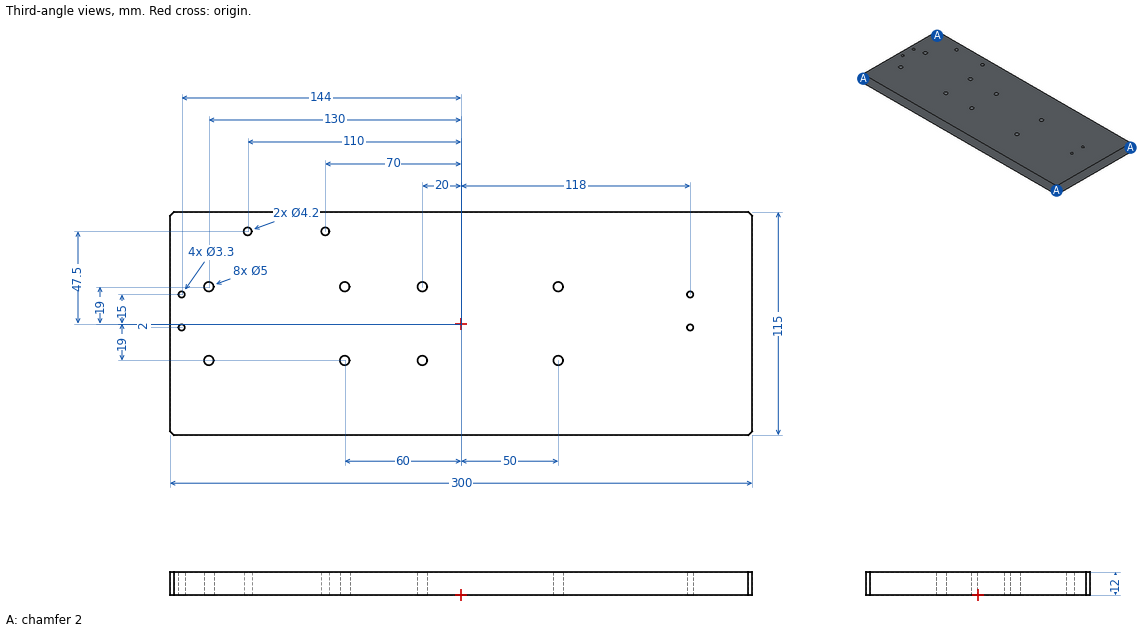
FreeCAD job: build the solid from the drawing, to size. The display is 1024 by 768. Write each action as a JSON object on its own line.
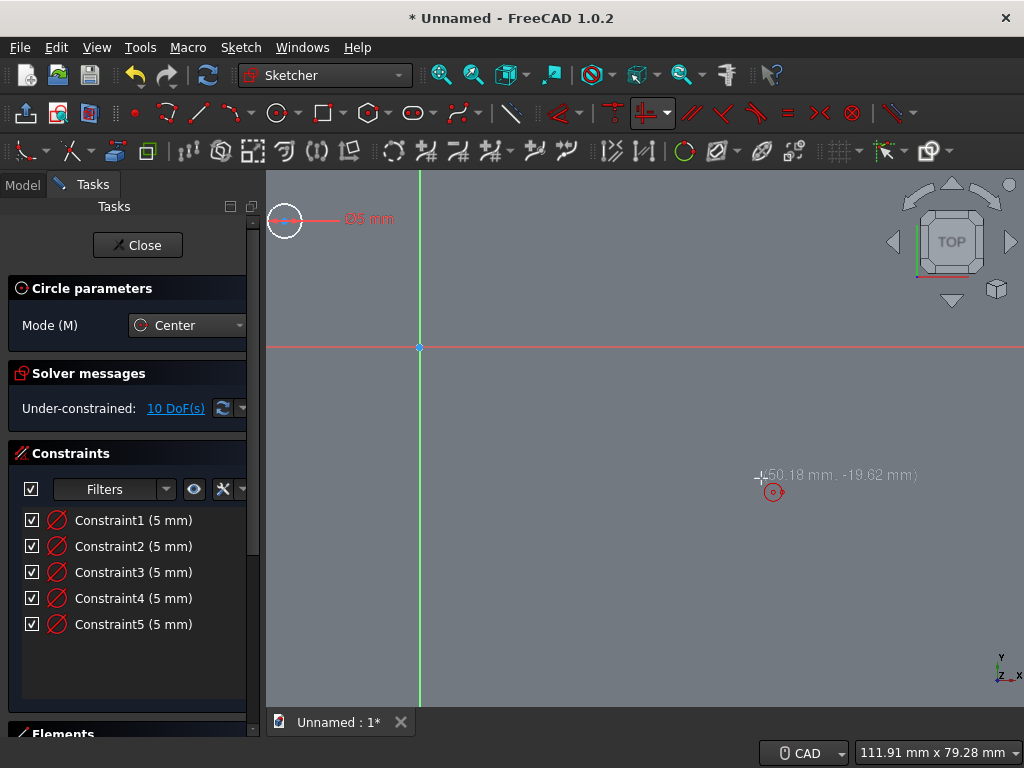
{"action": "scroll", "coordinate": [761, 478], "scroll_direction": "down", "scroll_amount": 8}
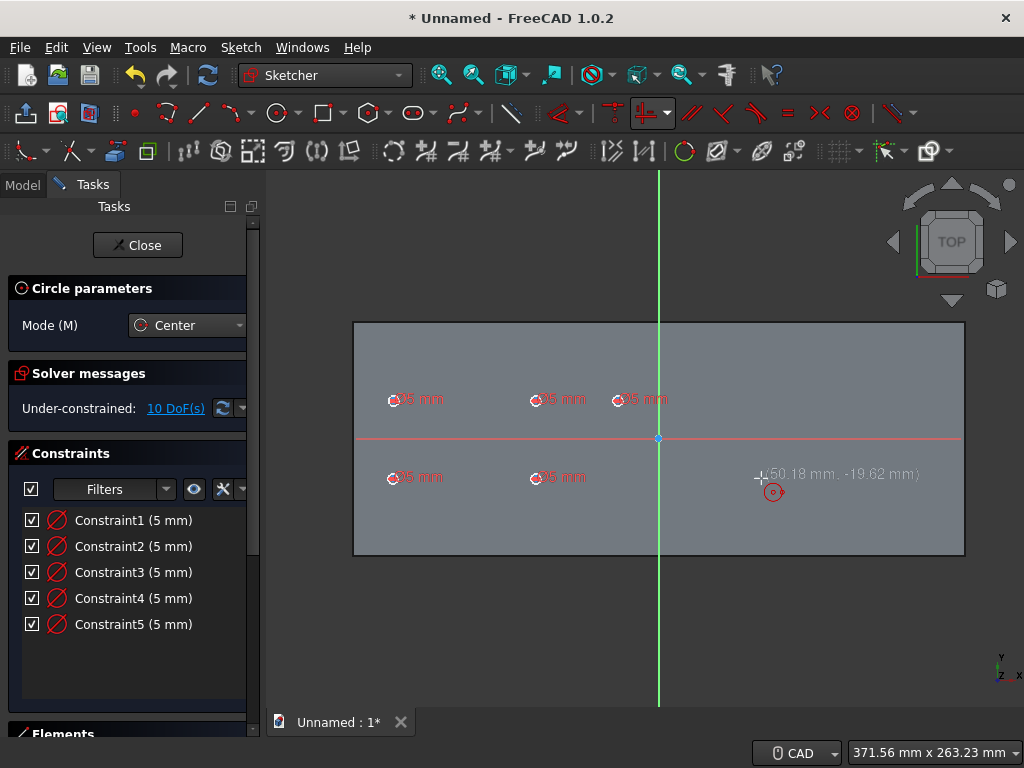
{"action": "left_click", "coordinate": [761, 478]}
{"action": "mouse_move", "coordinate": [764, 474]}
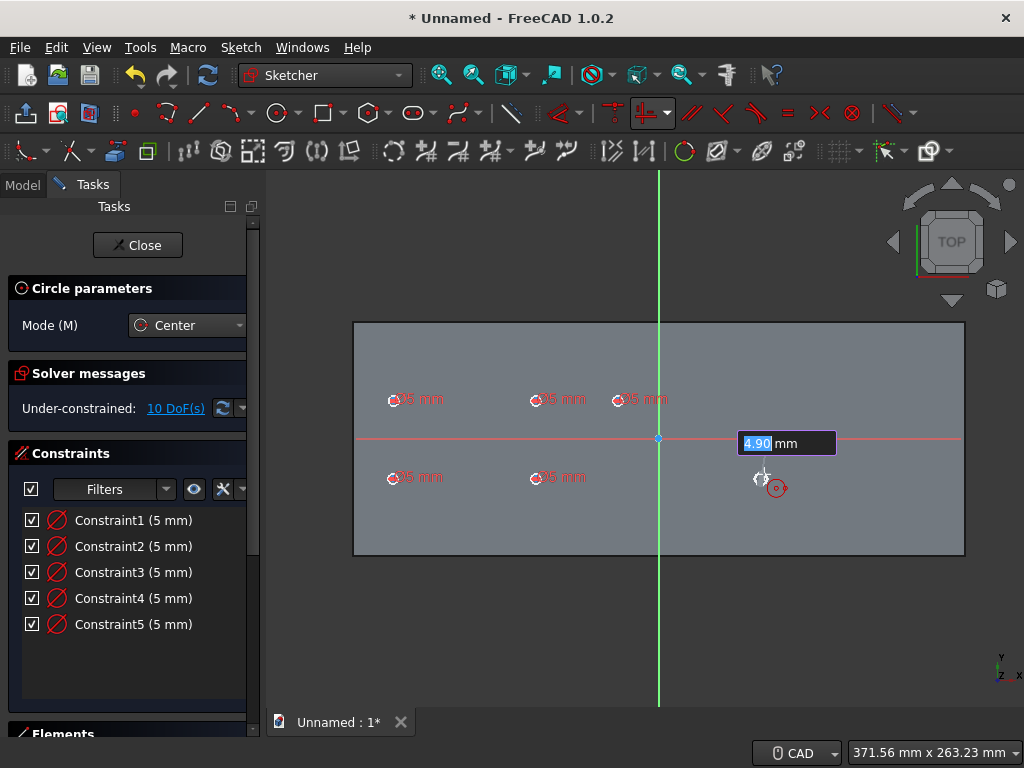
{"action": "type", "text": "5"}
{"action": "key", "text": "Return"}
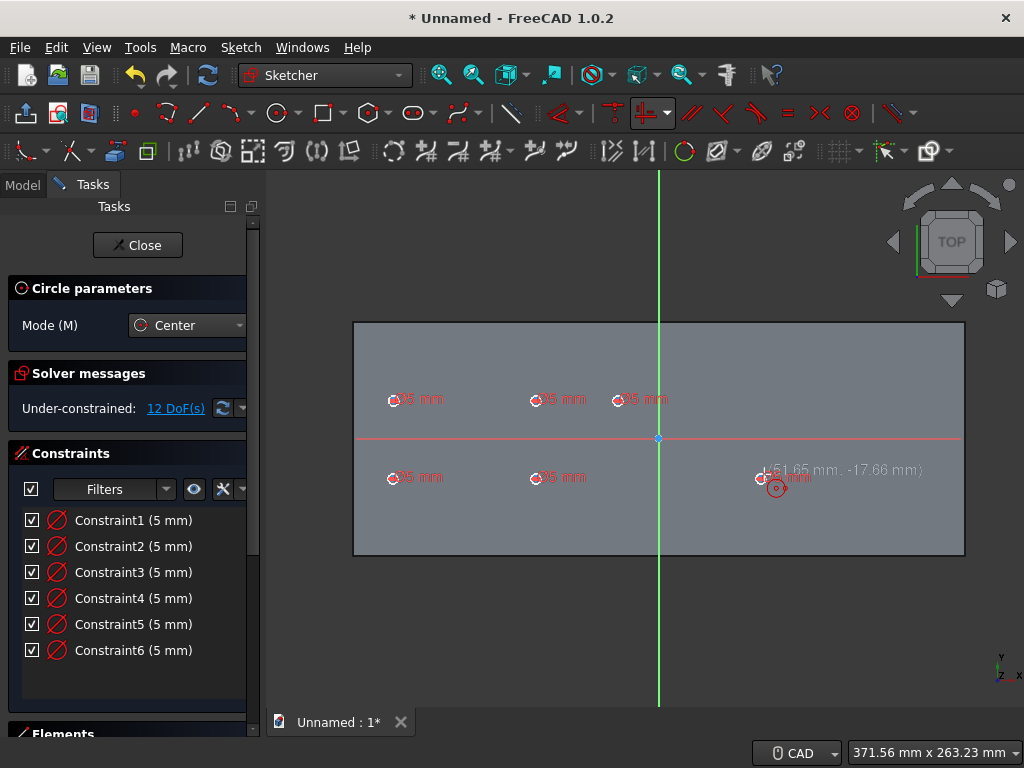
{"action": "scroll", "coordinate": [761, 400], "scroll_direction": "up", "scroll_amount": 8}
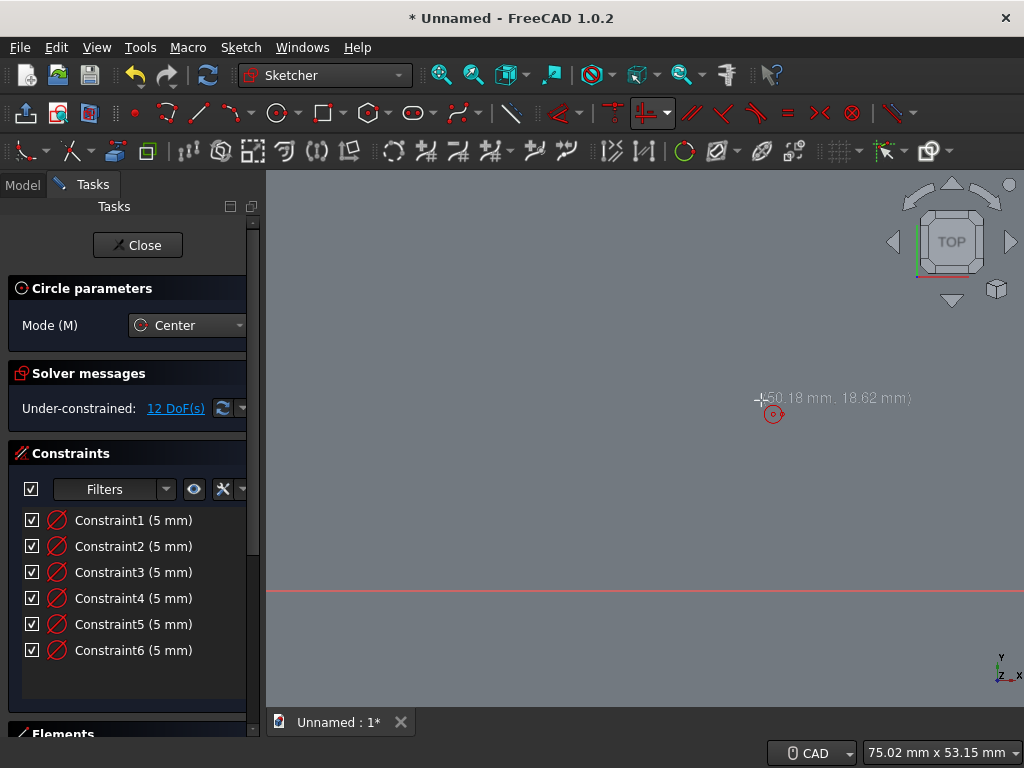
{"action": "scroll", "coordinate": [761, 400], "scroll_direction": "down", "scroll_amount": 8}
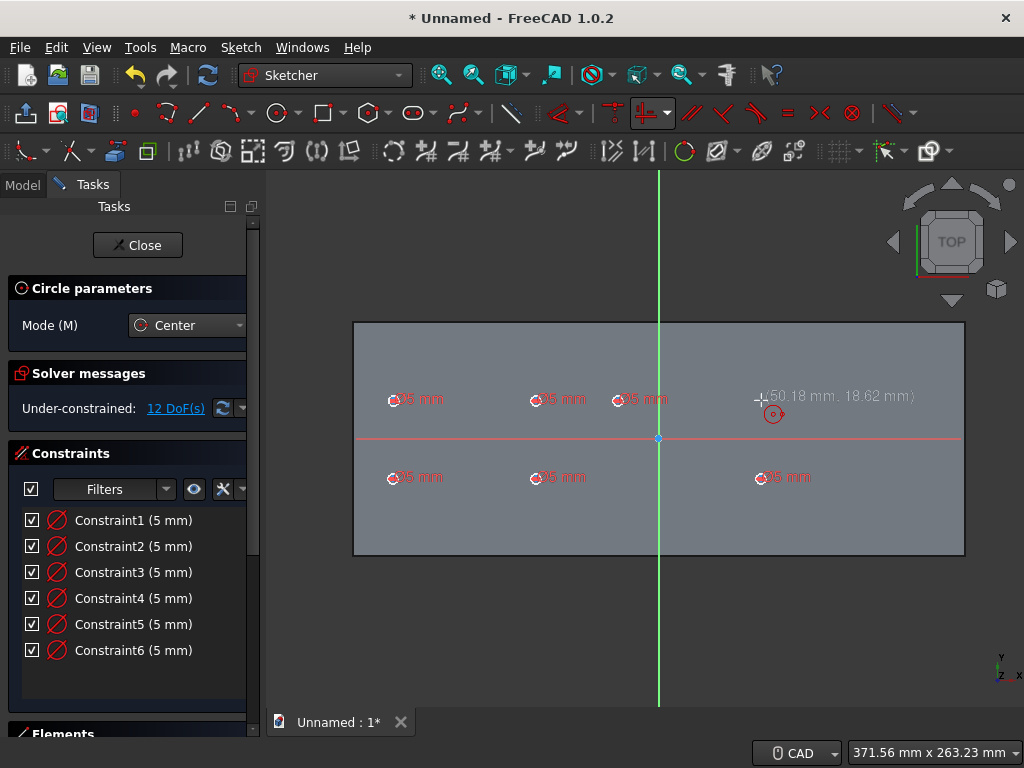
{"action": "left_click", "coordinate": [761, 400]}
{"action": "mouse_move", "coordinate": [764, 397]}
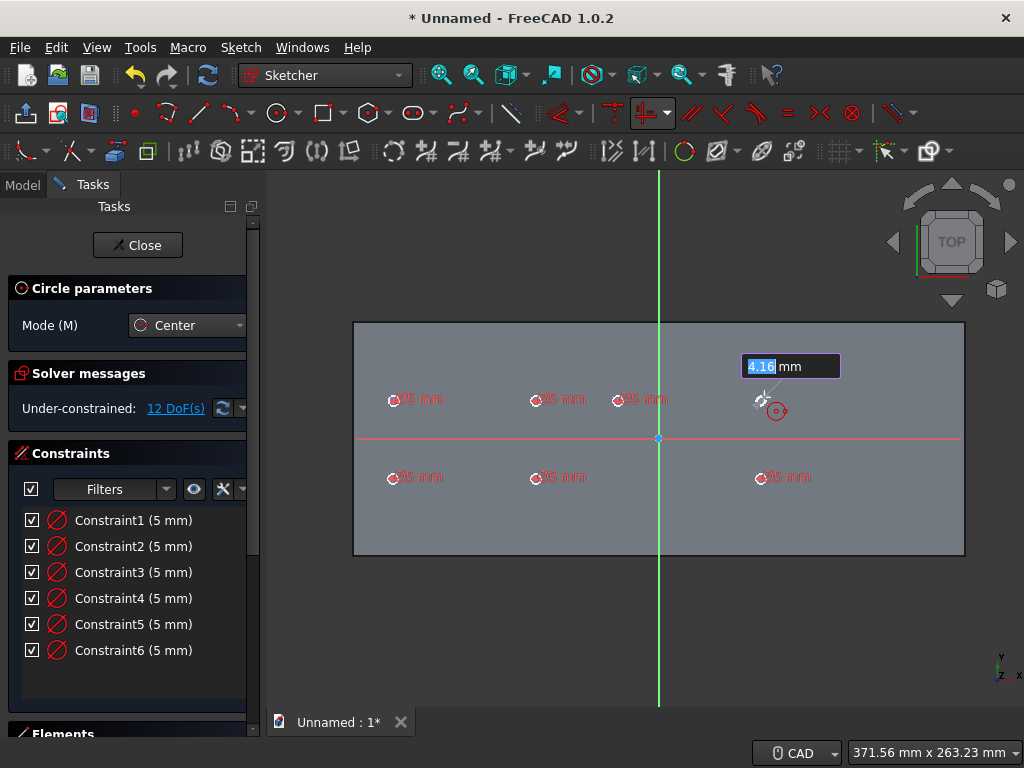
{"action": "type", "text": "5"}
{"action": "key", "text": "Return"}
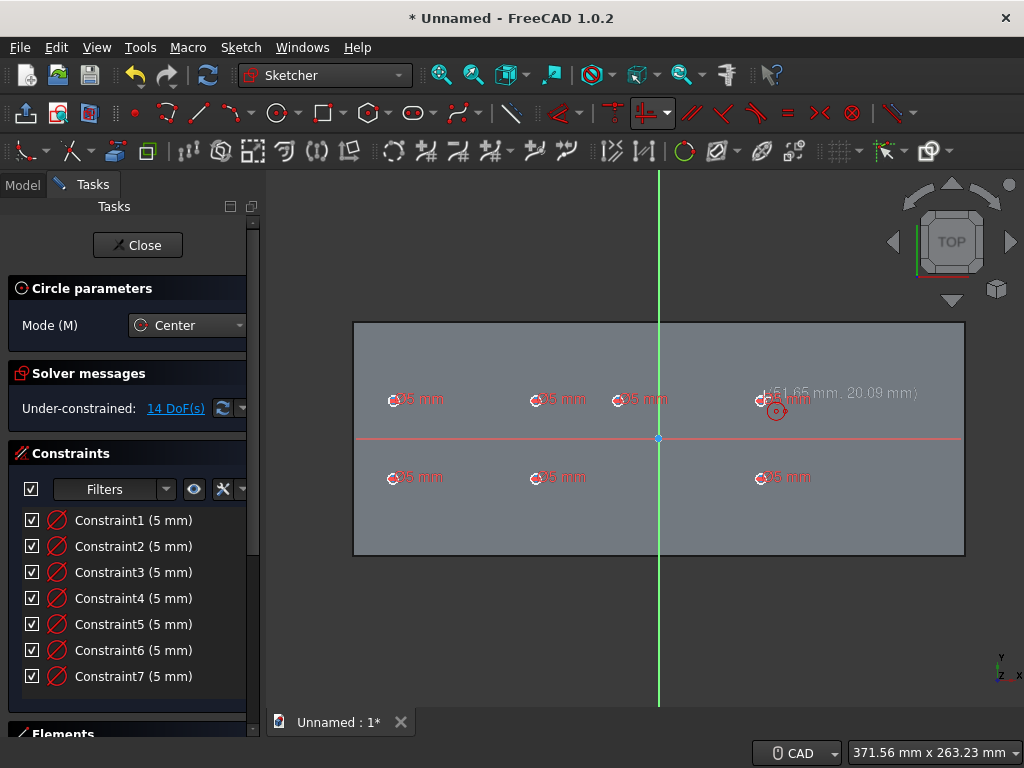
{"action": "scroll", "coordinate": [618, 478], "scroll_direction": "up", "scroll_amount": 8}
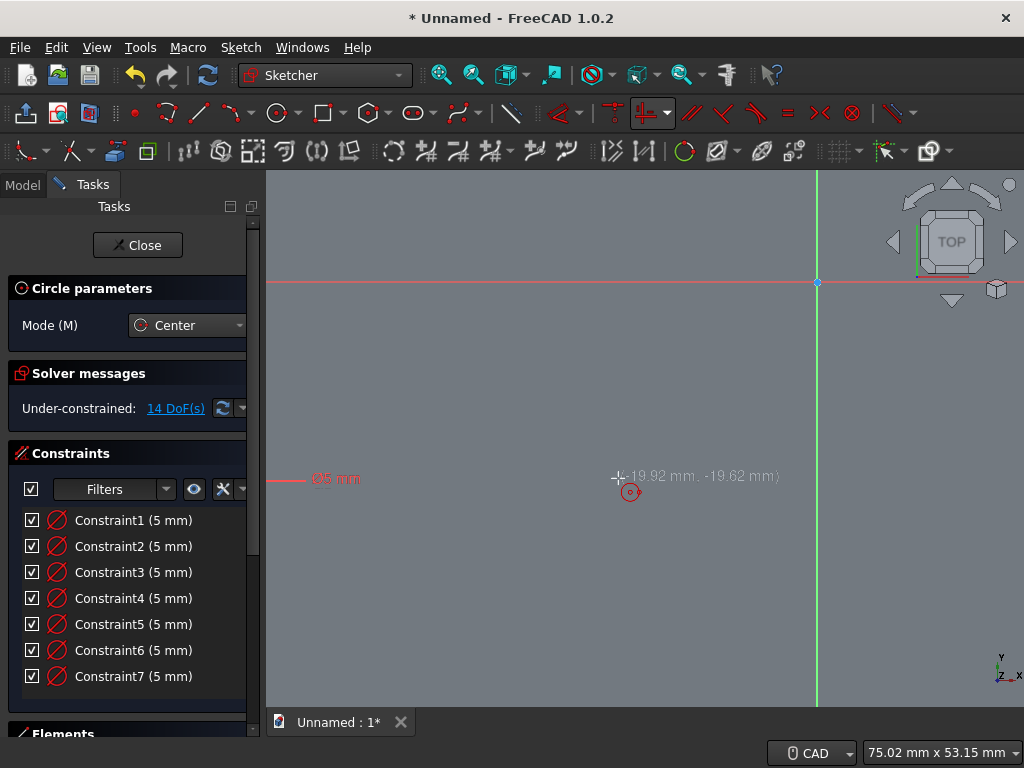
{"action": "scroll", "coordinate": [618, 478], "scroll_direction": "down", "scroll_amount": 8}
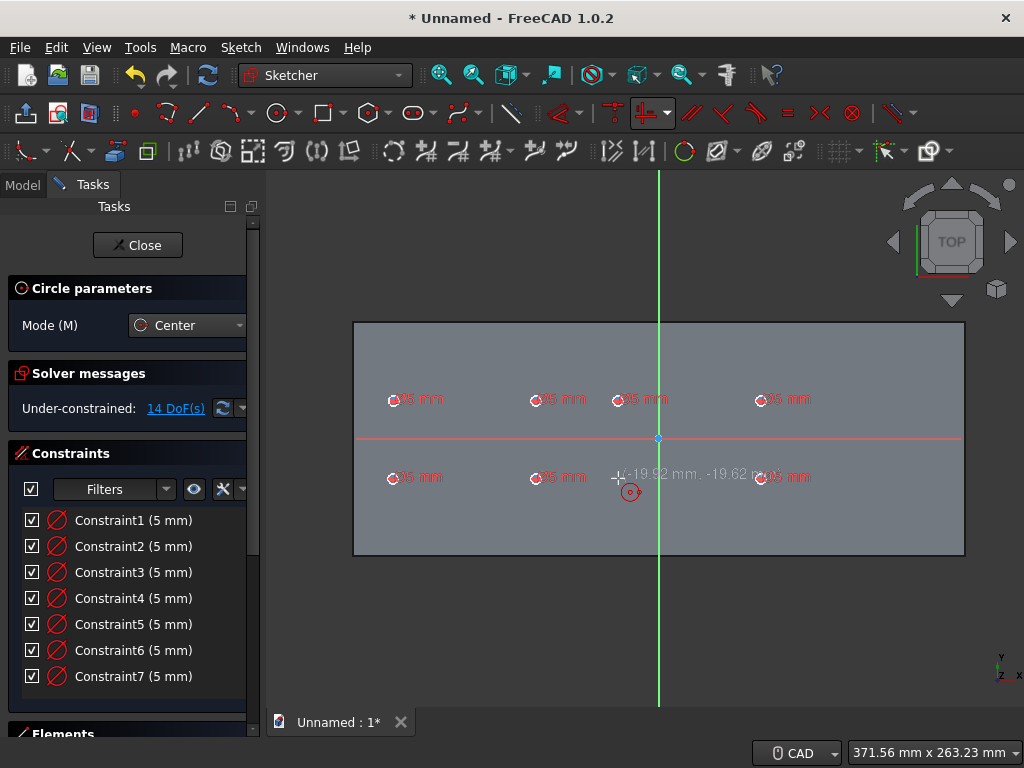
{"action": "left_click", "coordinate": [618, 478]}
{"action": "mouse_move", "coordinate": [621, 474]}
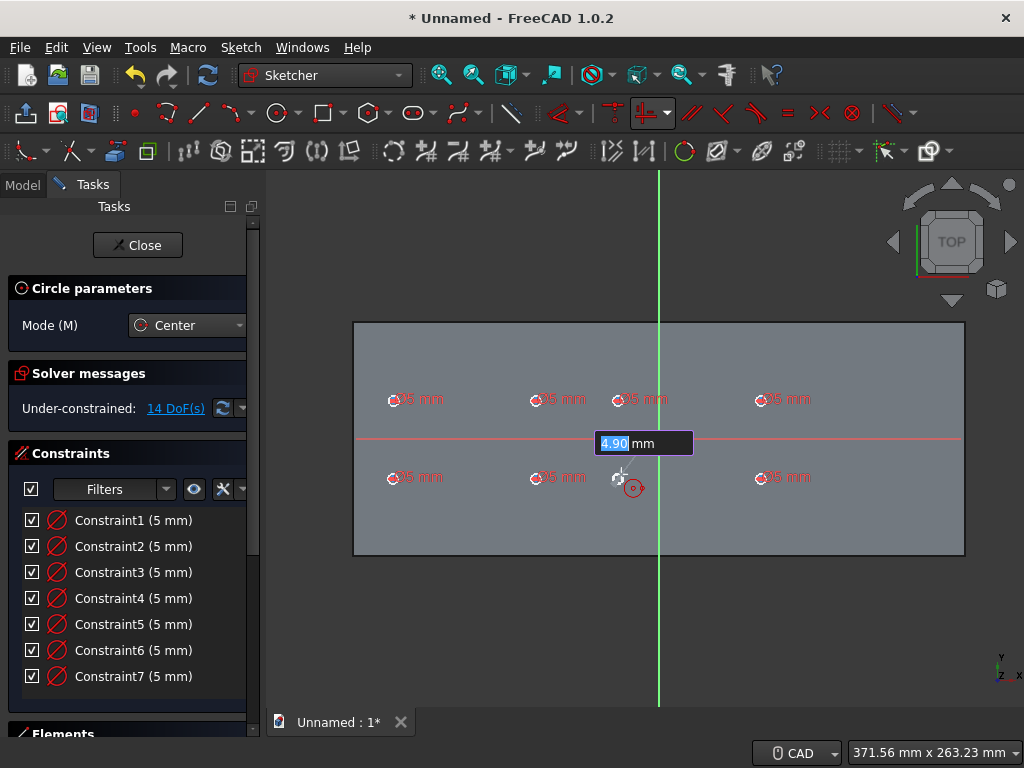
{"action": "type", "text": "5"}
{"action": "key", "text": "Return"}
{"action": "key", "text": "Escape"}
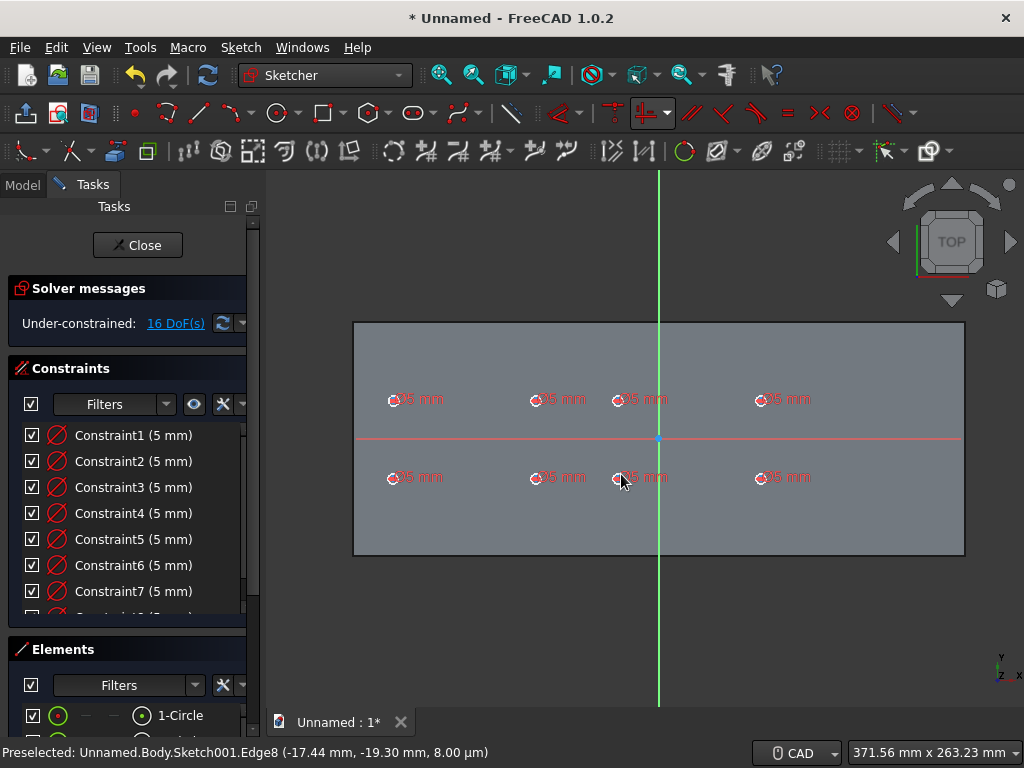
{"action": "left_click", "coordinate": [536, 479]}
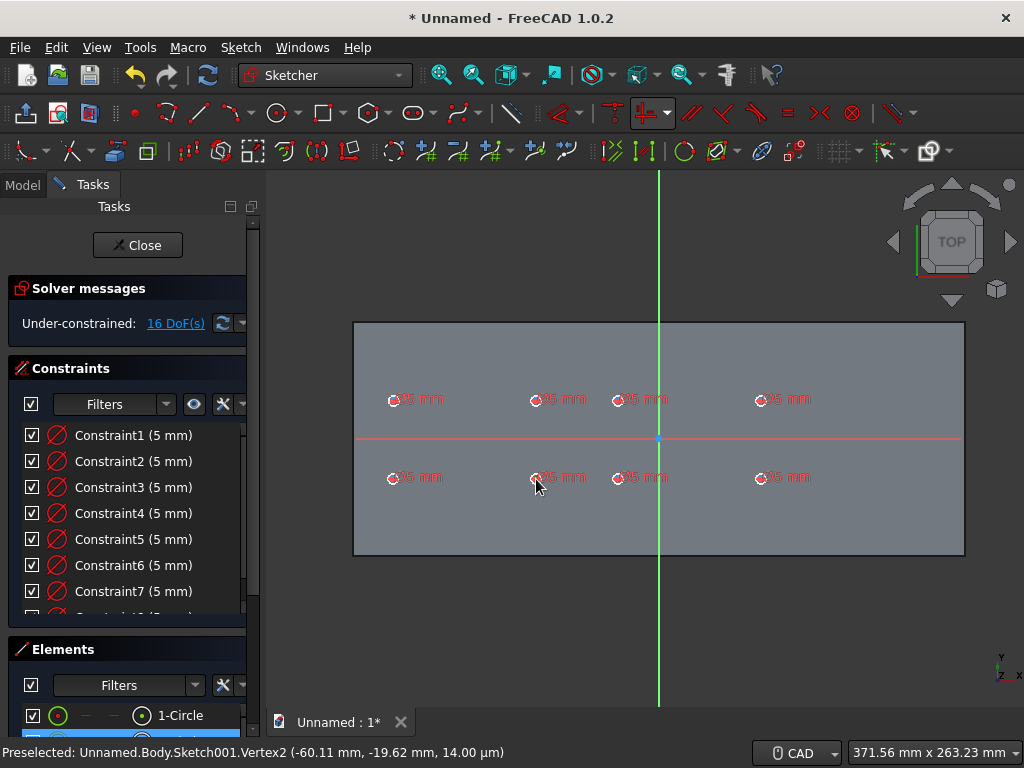
{"action": "left_click", "coordinate": [536, 401]}